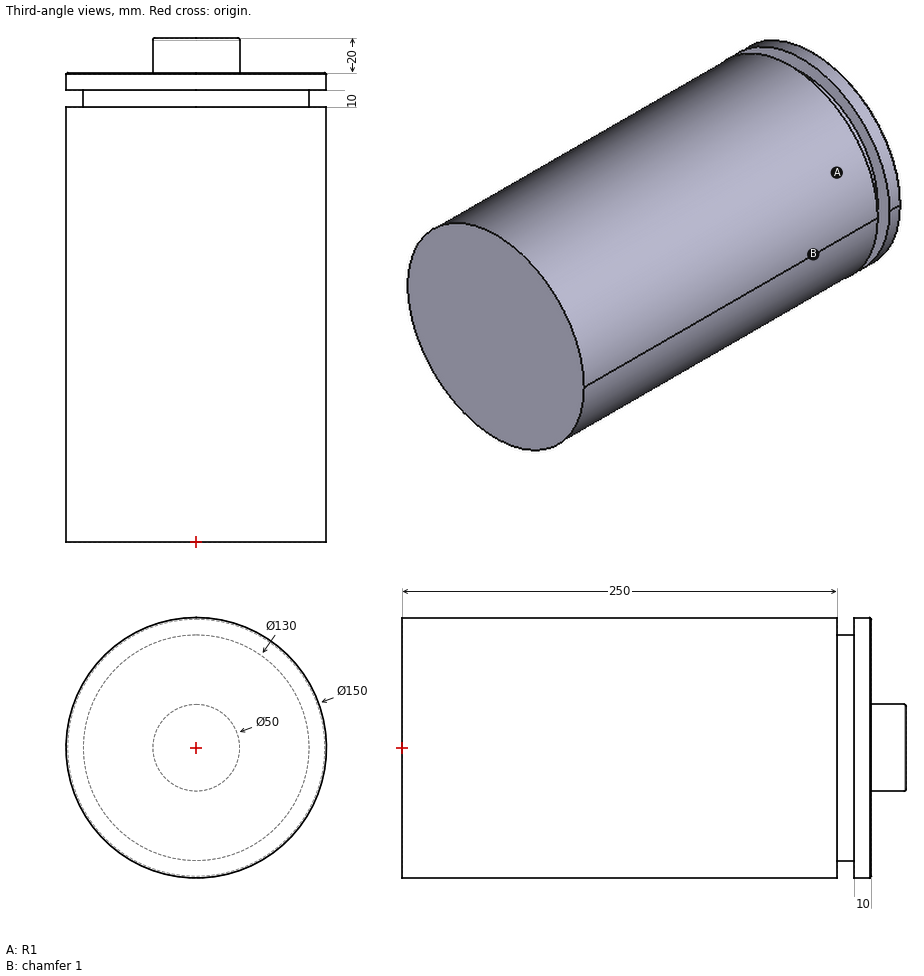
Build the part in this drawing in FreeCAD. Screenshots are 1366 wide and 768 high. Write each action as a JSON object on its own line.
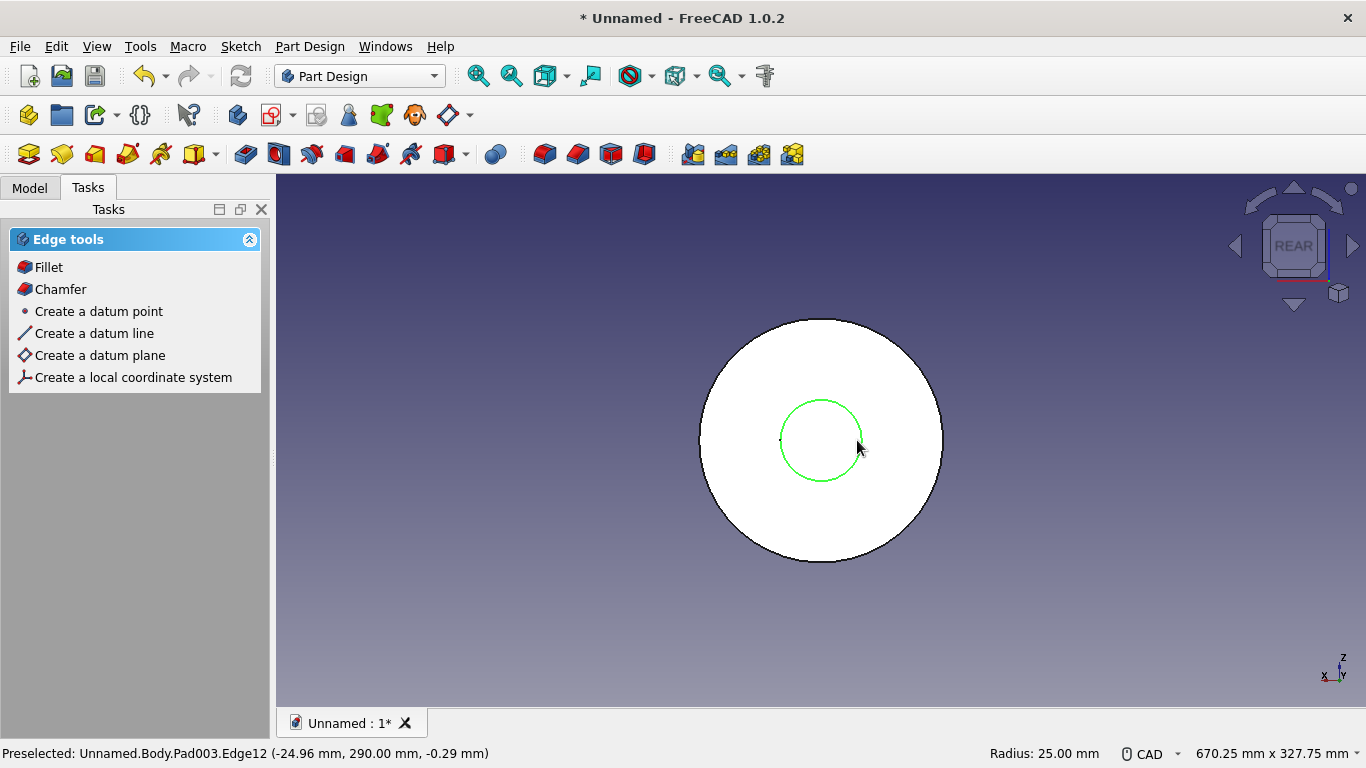
{"action": "left_click", "coordinate": [545, 154]}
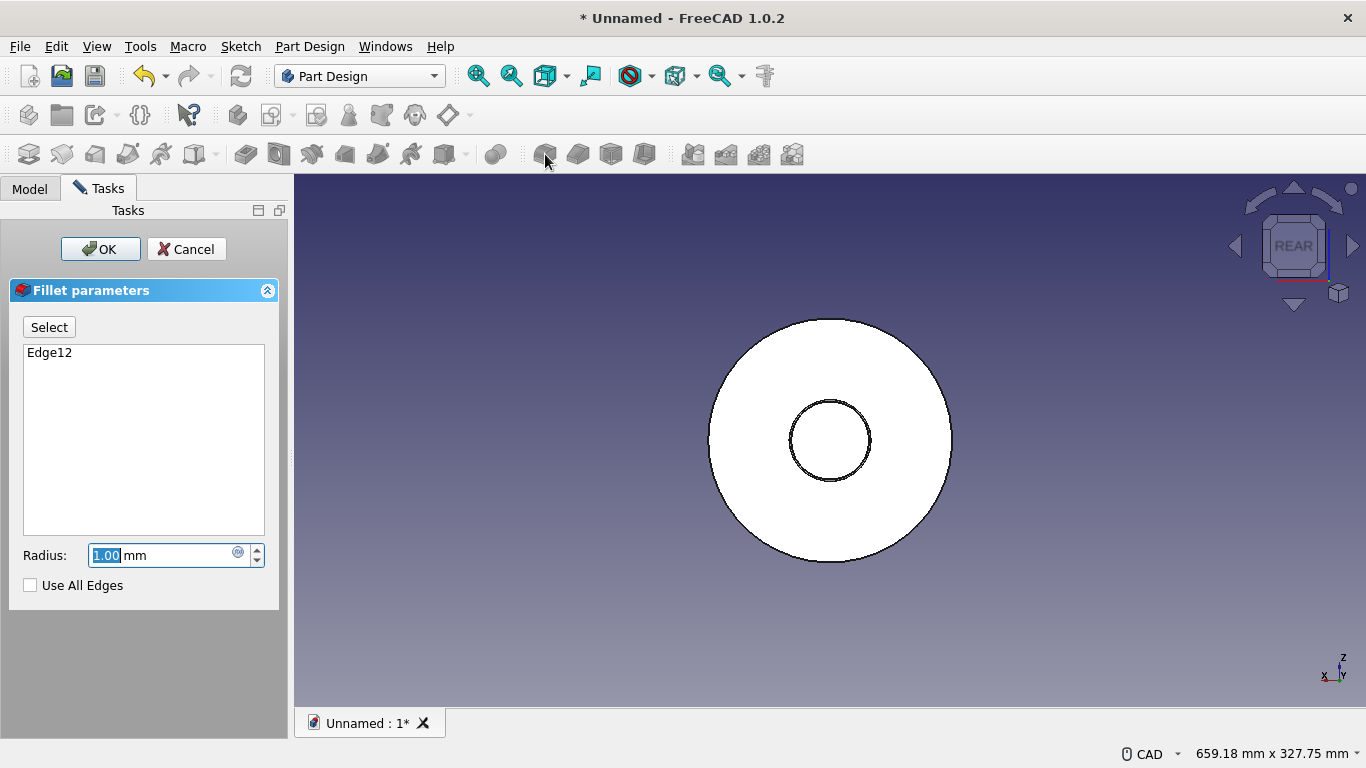
{"action": "type", "text": "1"}
{"action": "key", "text": "Tab"}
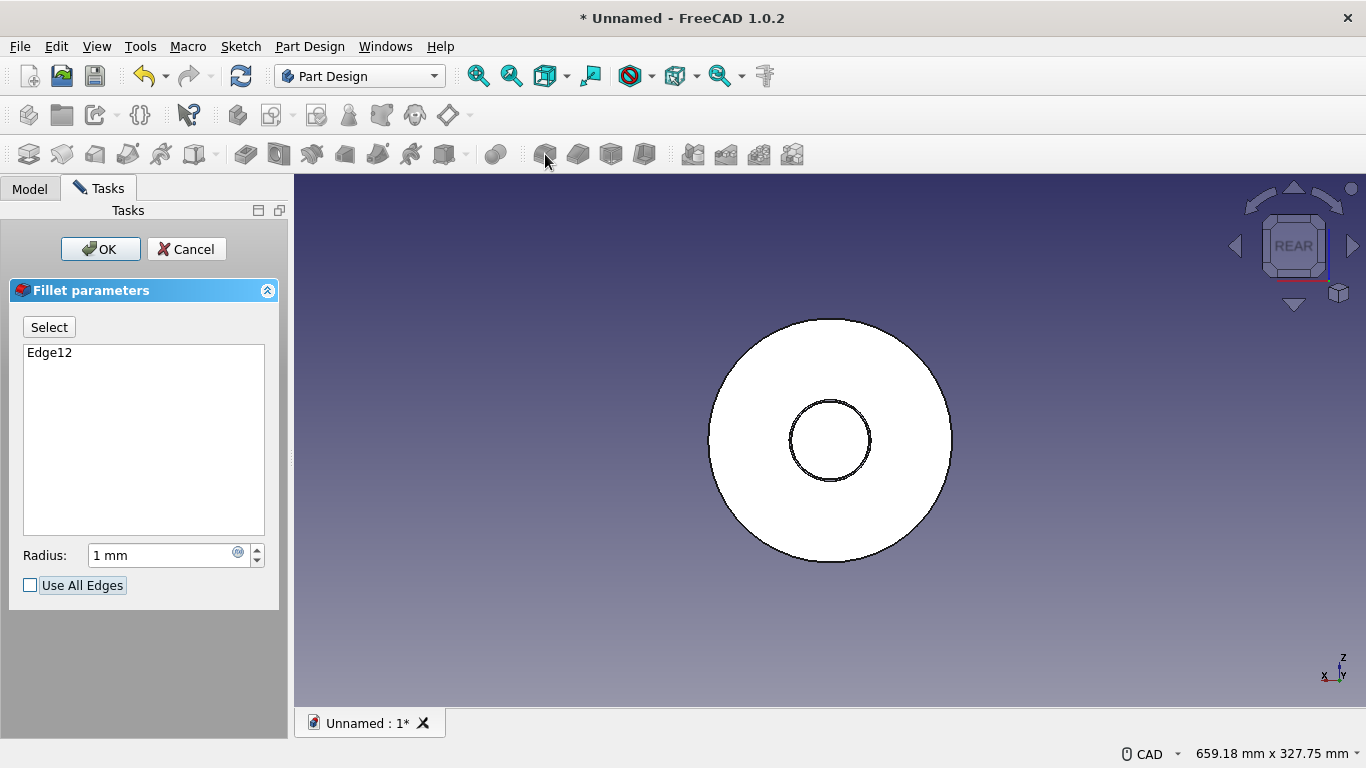
{"action": "left_click", "coordinate": [101, 249]}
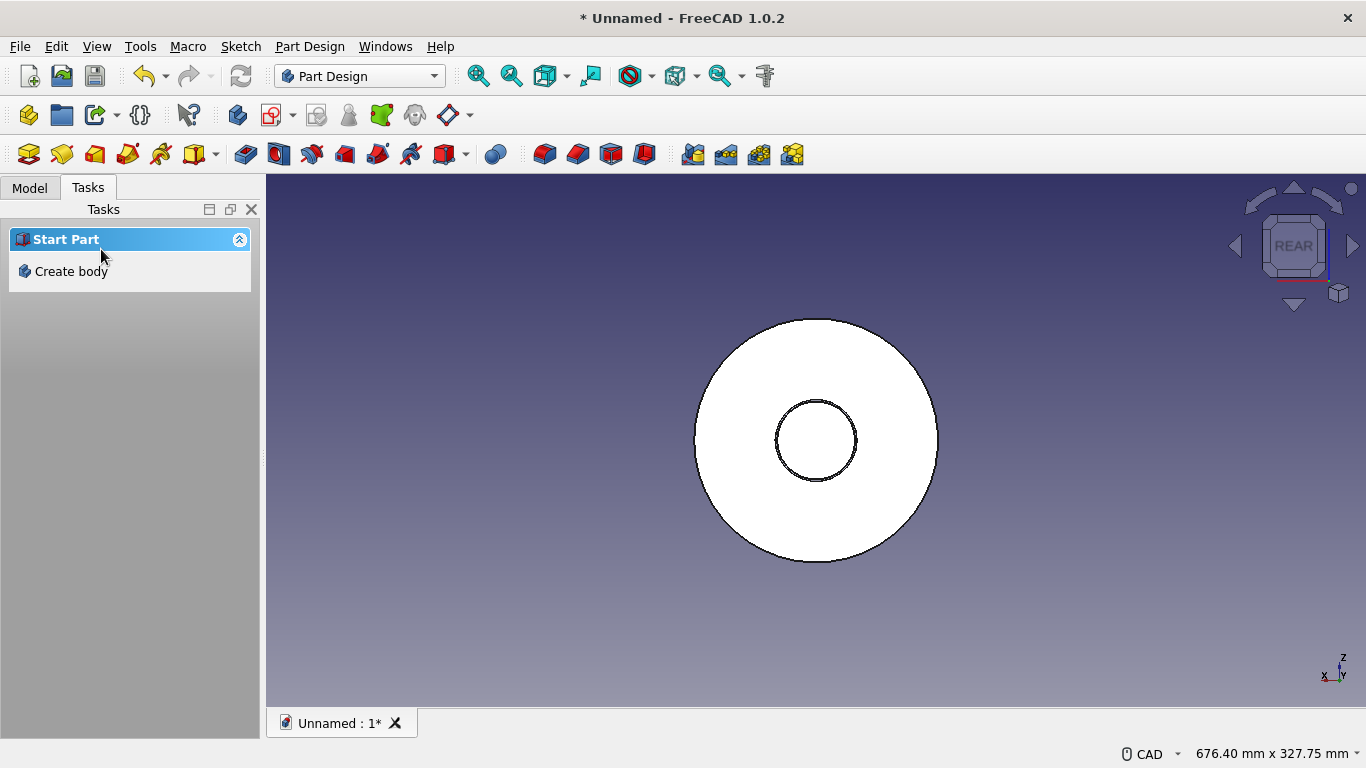
{"action": "left_click", "coordinate": [938, 440]}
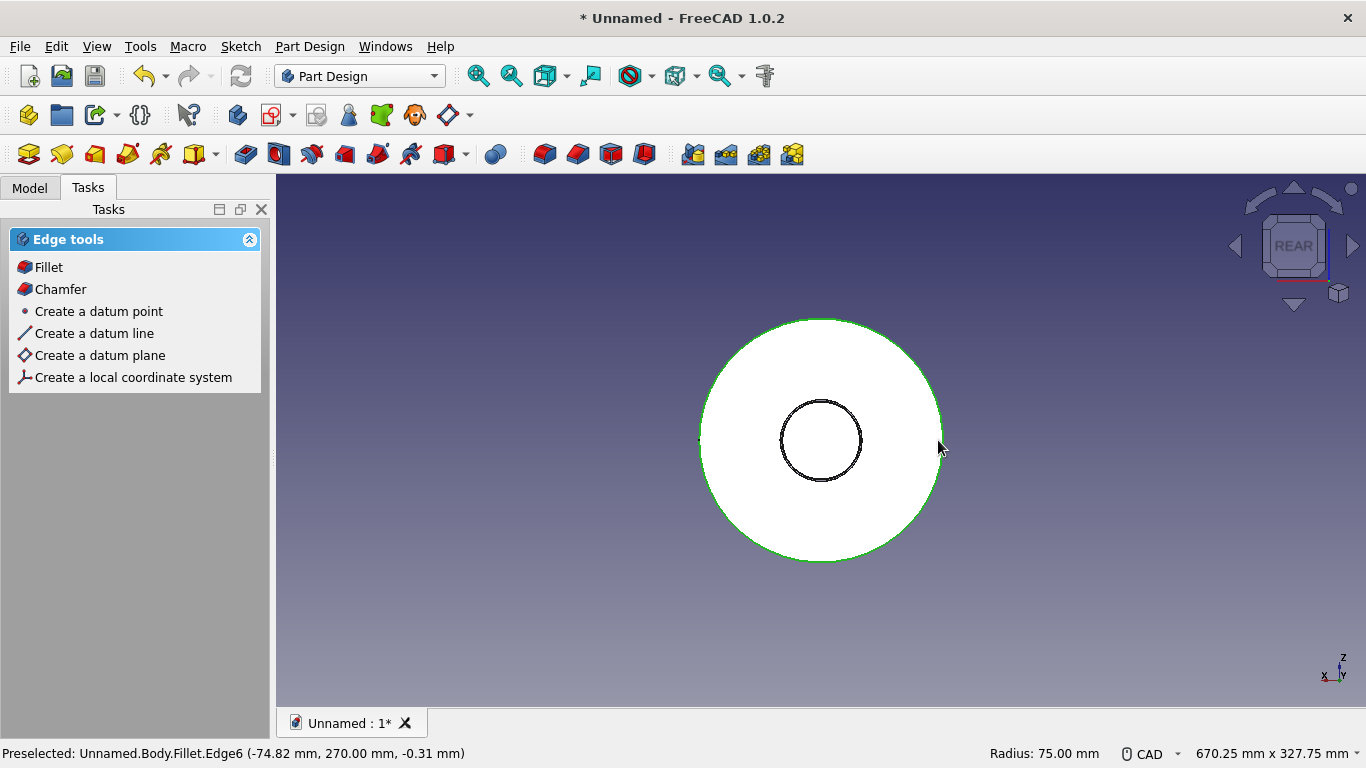
{"action": "left_click", "coordinate": [578, 154]}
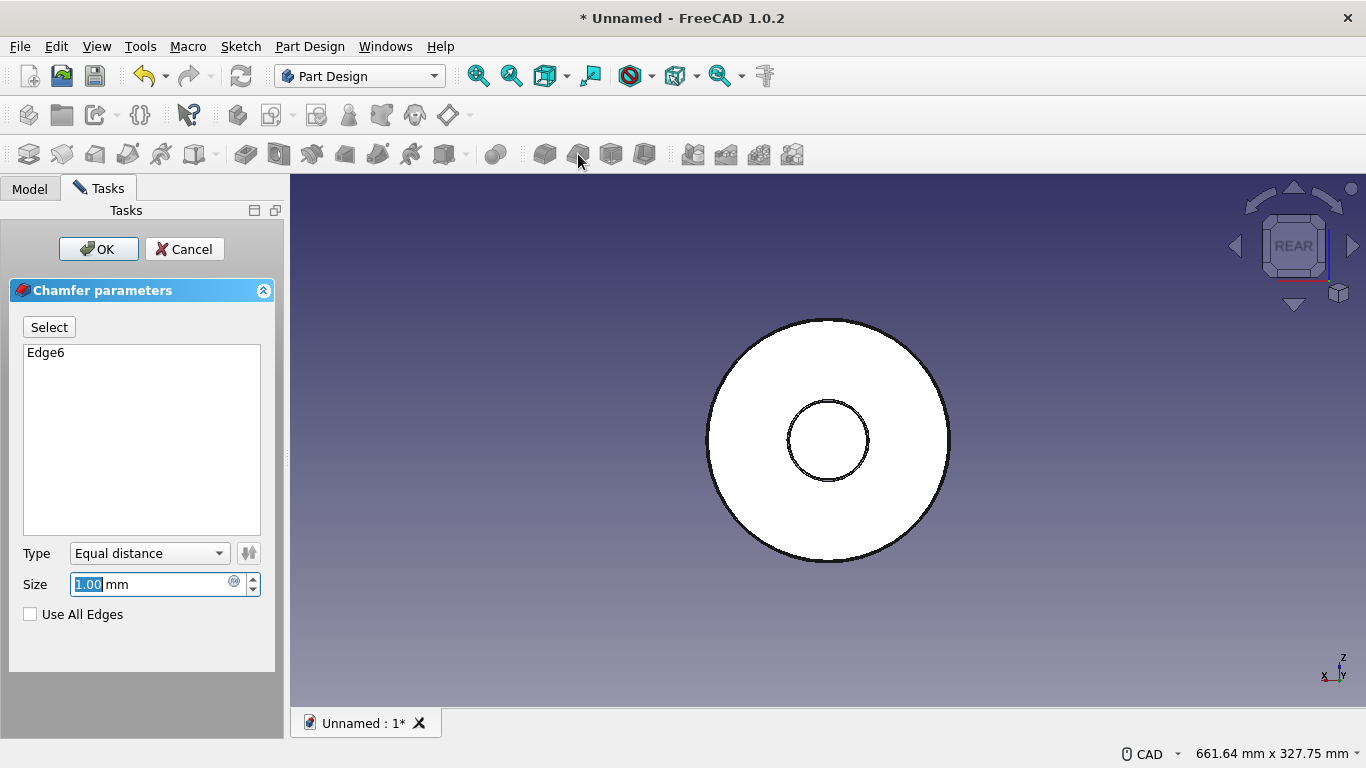
{"action": "type", "text": "1"}
{"action": "key", "text": "Tab"}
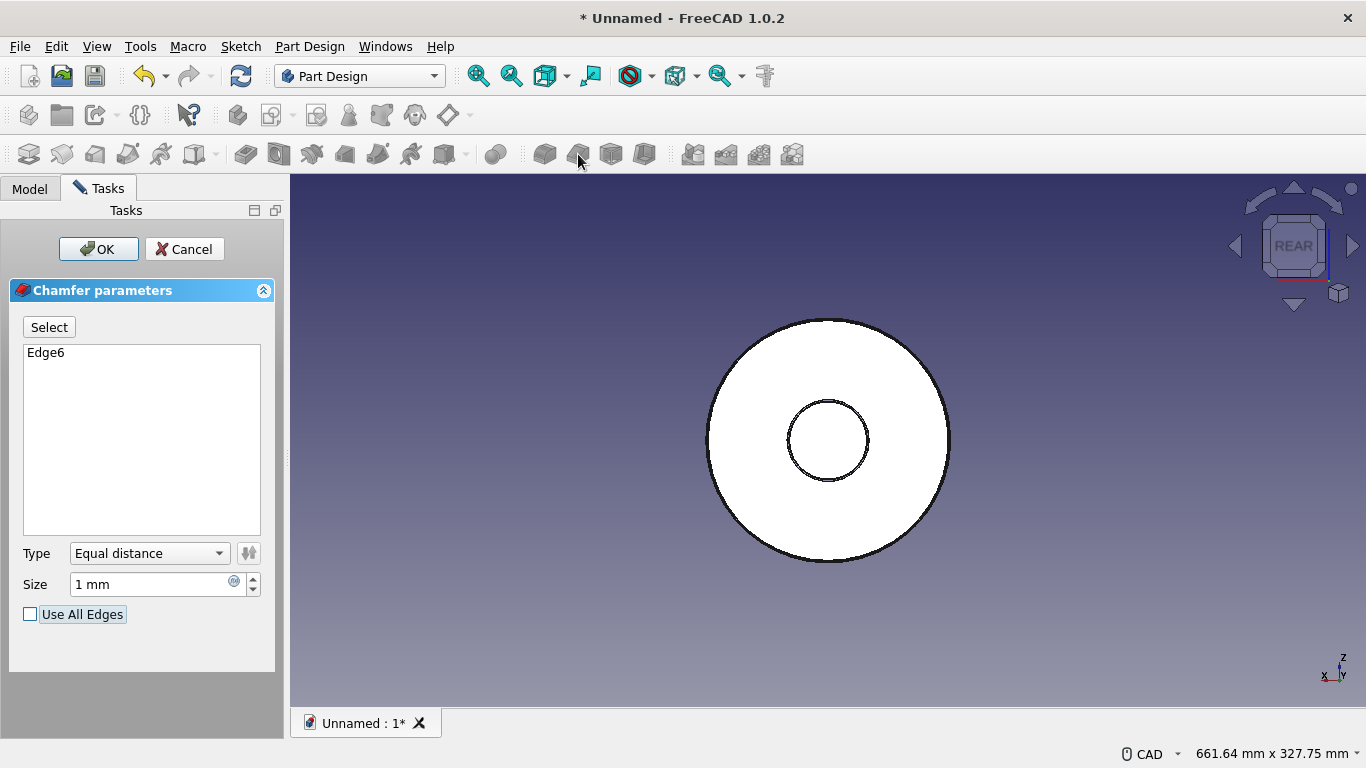
{"action": "left_click", "coordinate": [99, 249]}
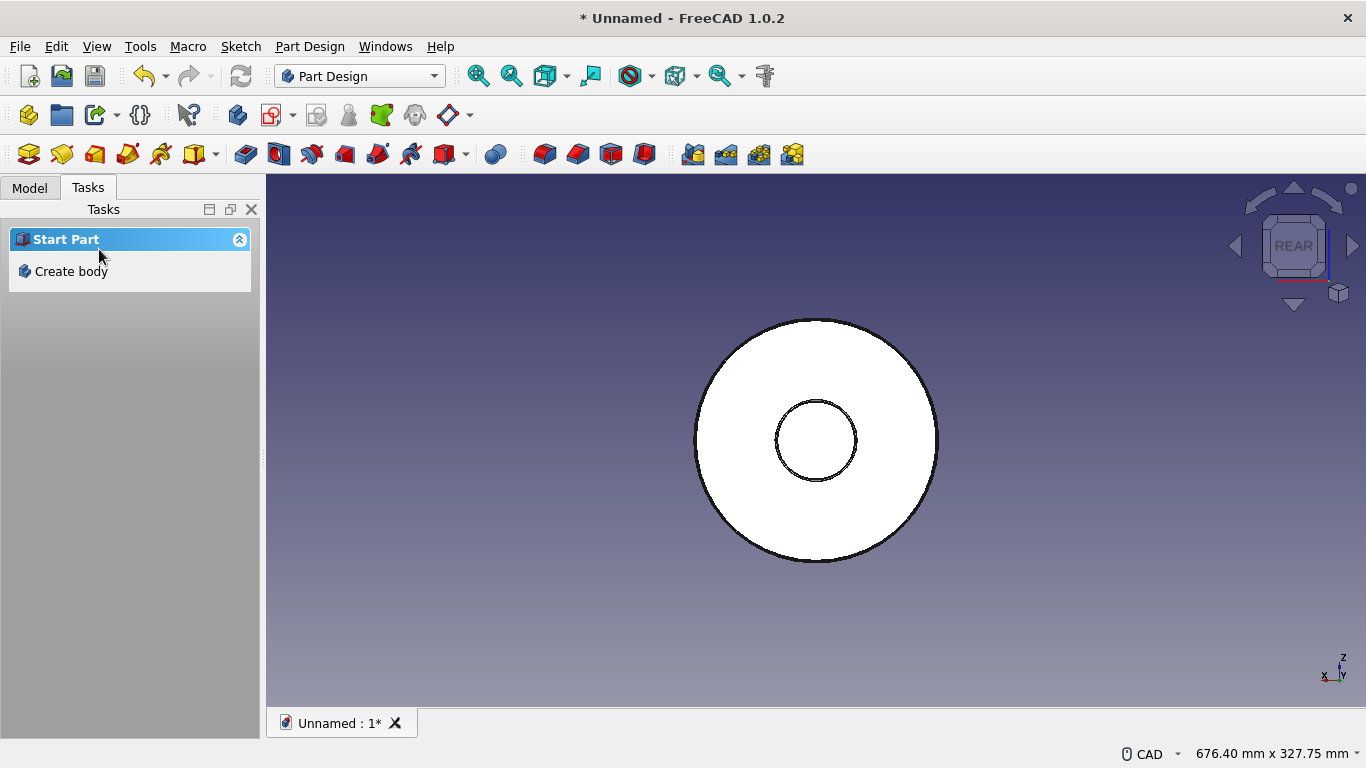
{"action": "key", "text": "0"}